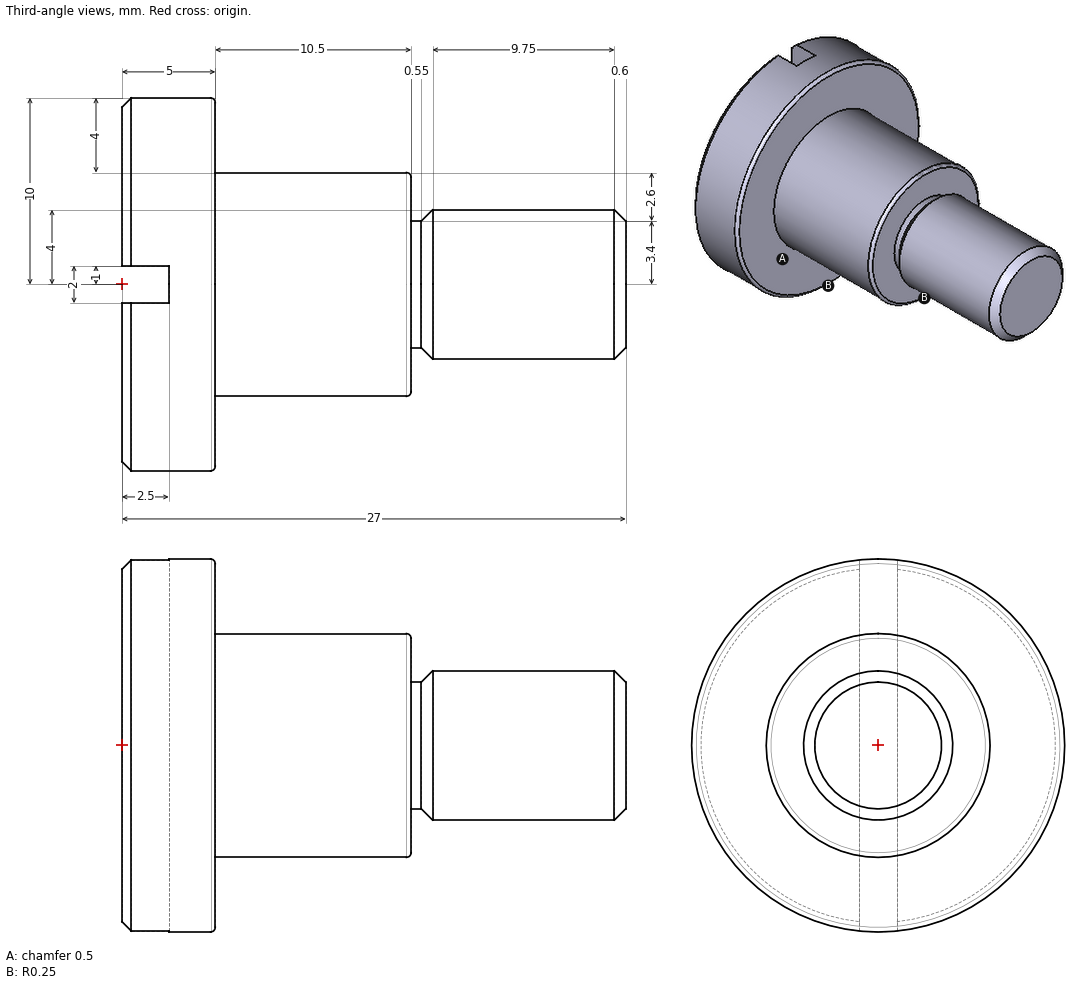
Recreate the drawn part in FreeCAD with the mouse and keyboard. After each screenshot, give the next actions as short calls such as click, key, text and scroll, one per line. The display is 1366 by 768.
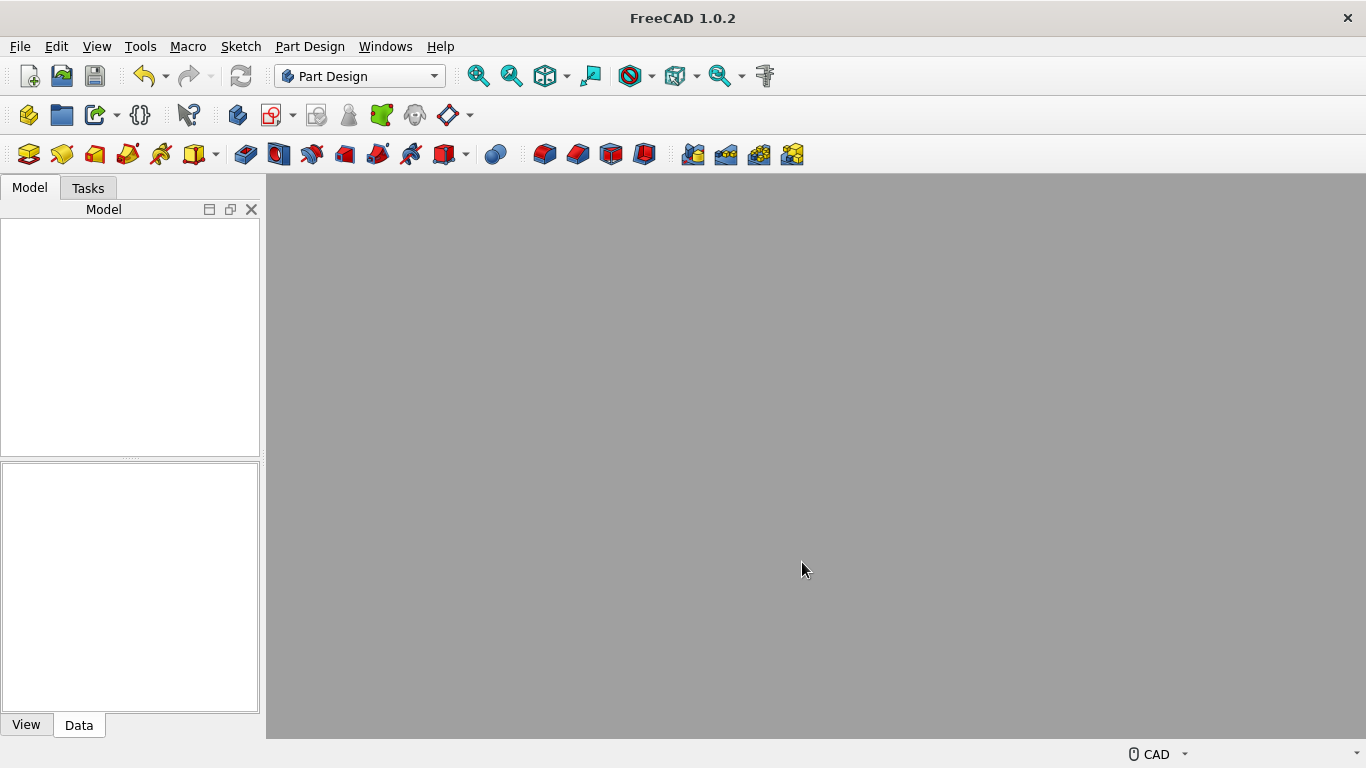
click(29, 76)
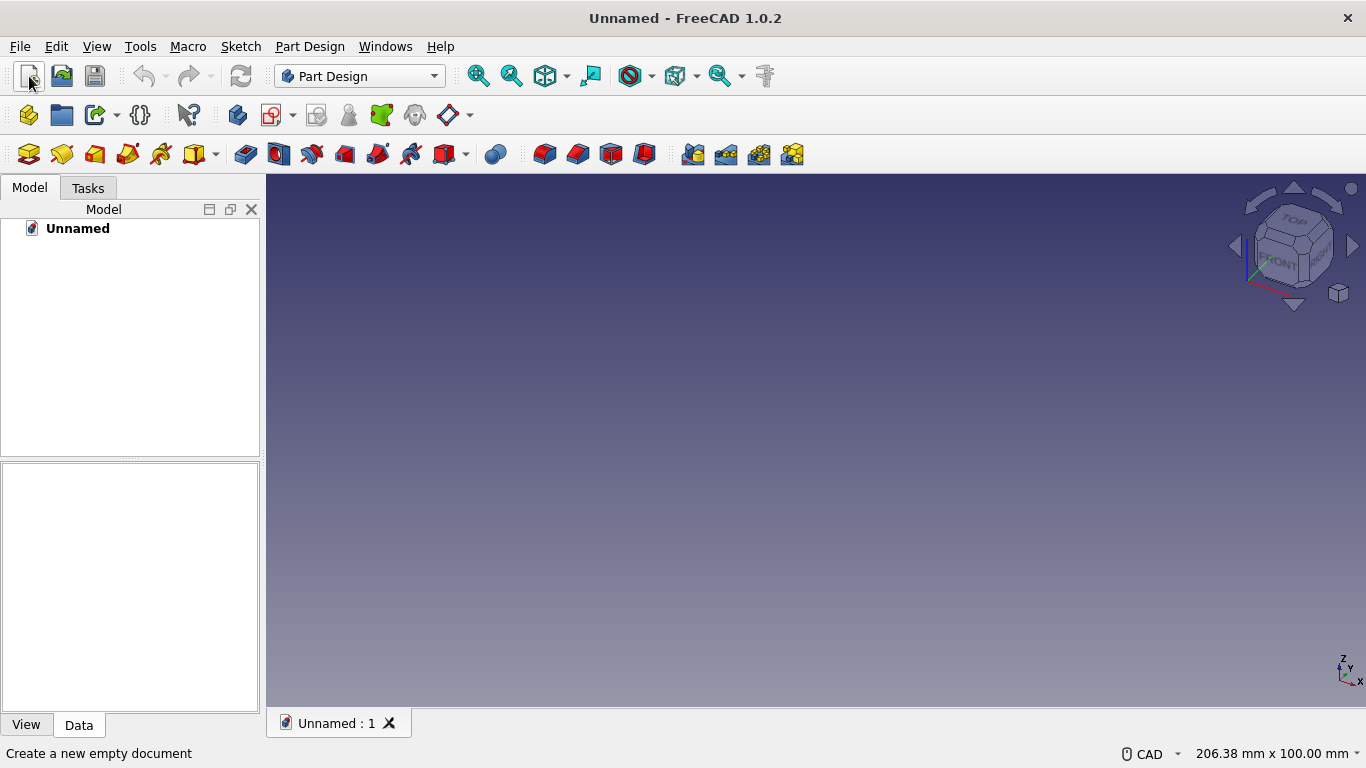
click(270, 116)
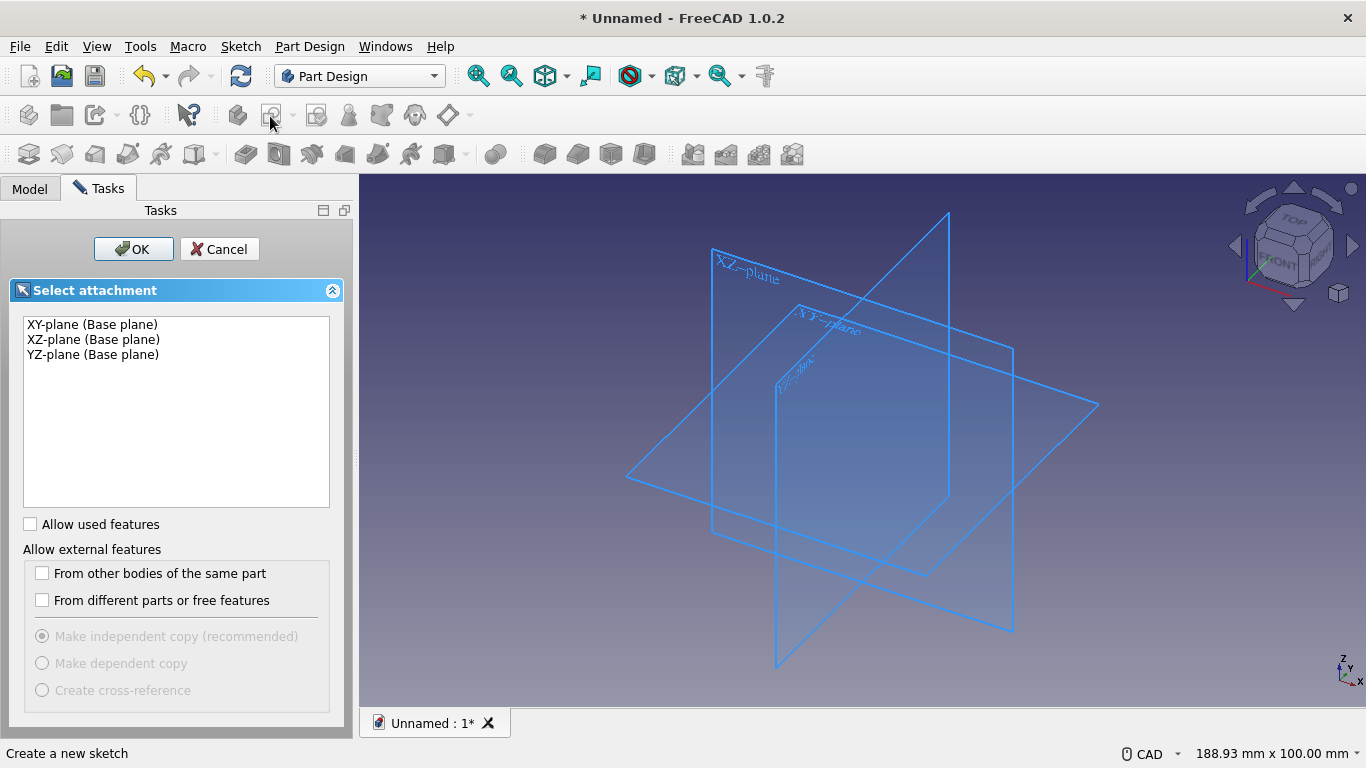
click(84, 324)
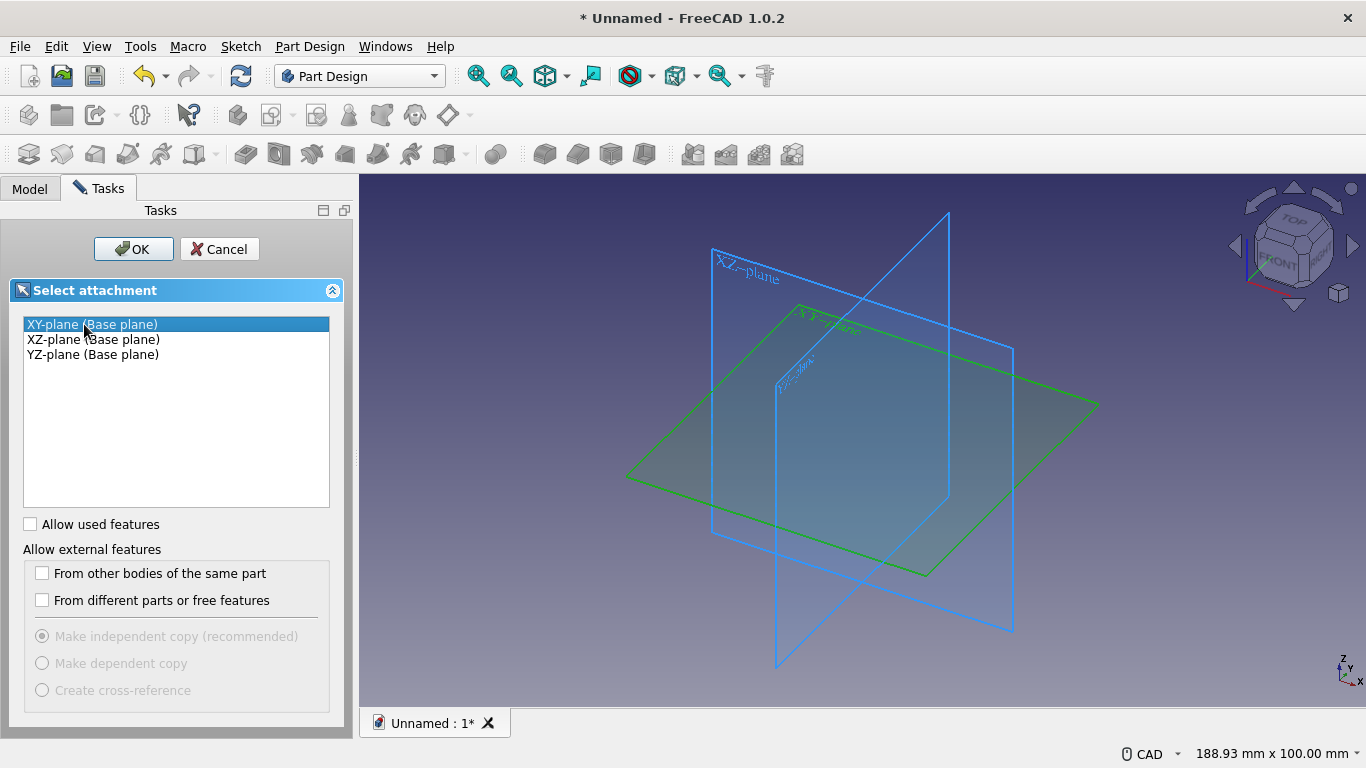
click(134, 249)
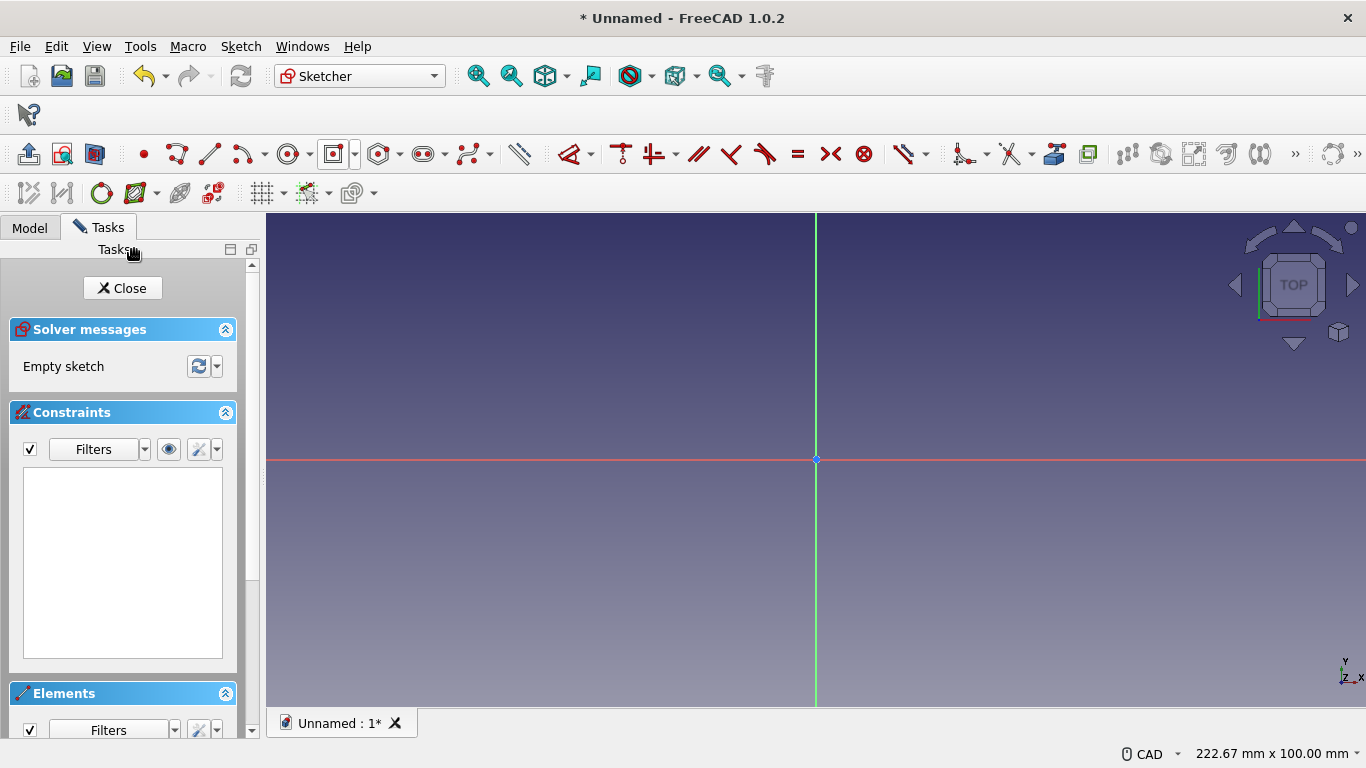
scroll(917, 429, up, 8)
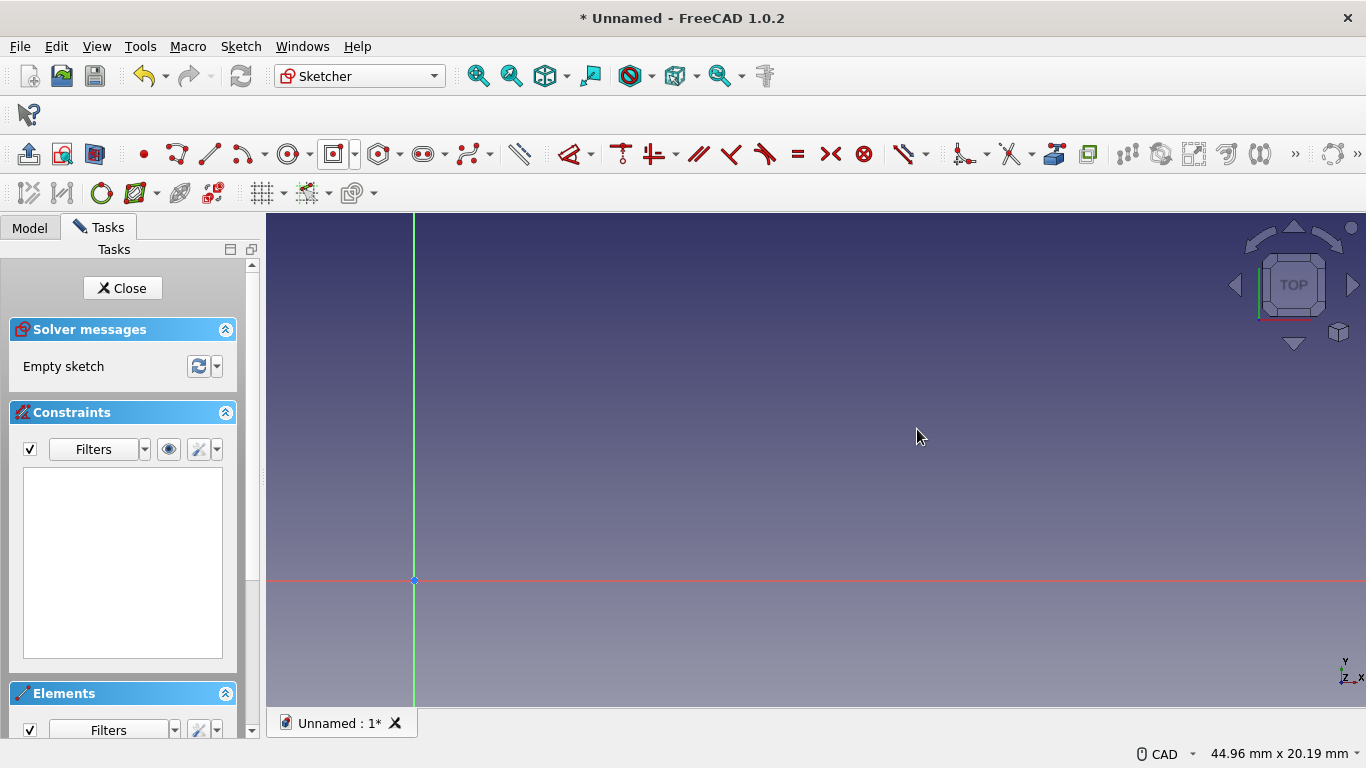
click(177, 154)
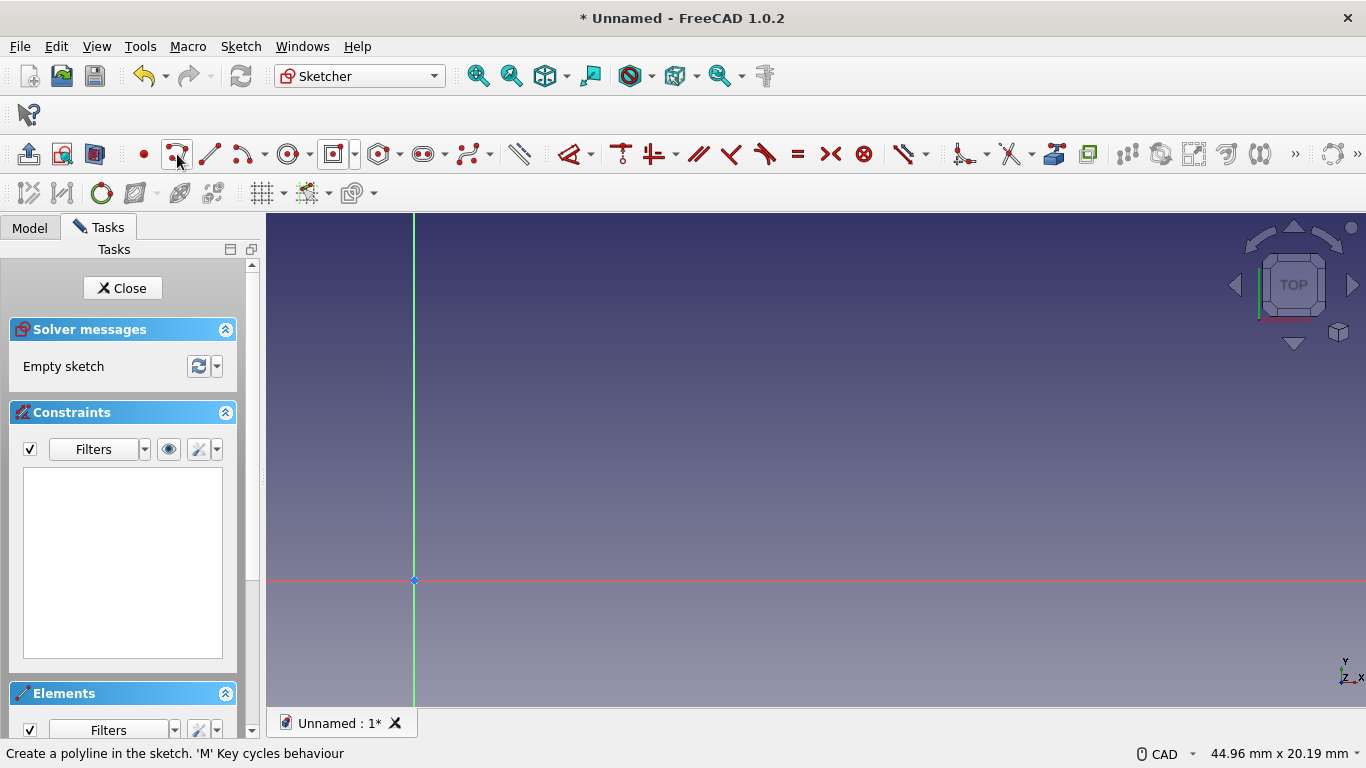
click(414, 581)
click(1075, 572)
click(1075, 498)
click(1060, 483)
click(822, 483)
click(807, 498)
click(794, 498)
click(794, 434)
click(537, 434)
click(537, 336)
click(423, 336)
click(414, 581)
key(Escape)
key(Escape)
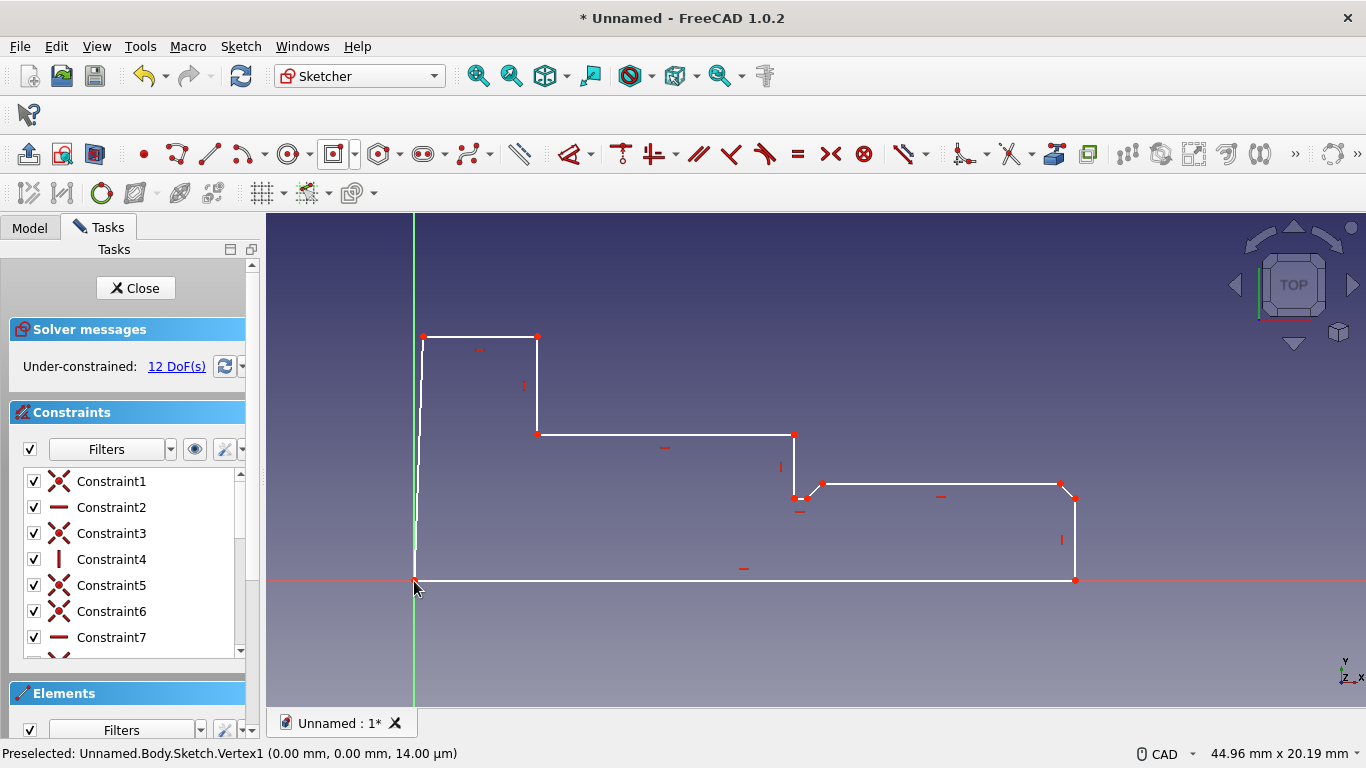
click(417, 508)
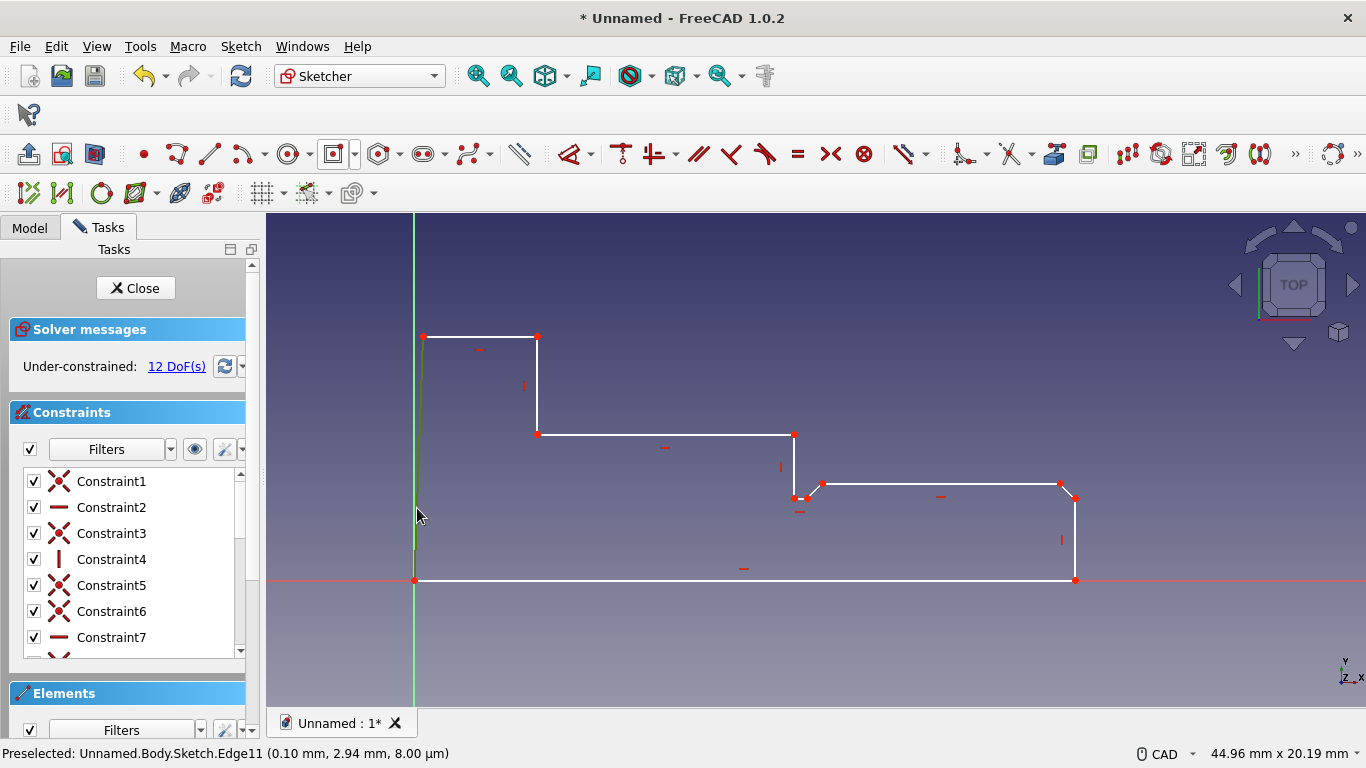
click(676, 154)